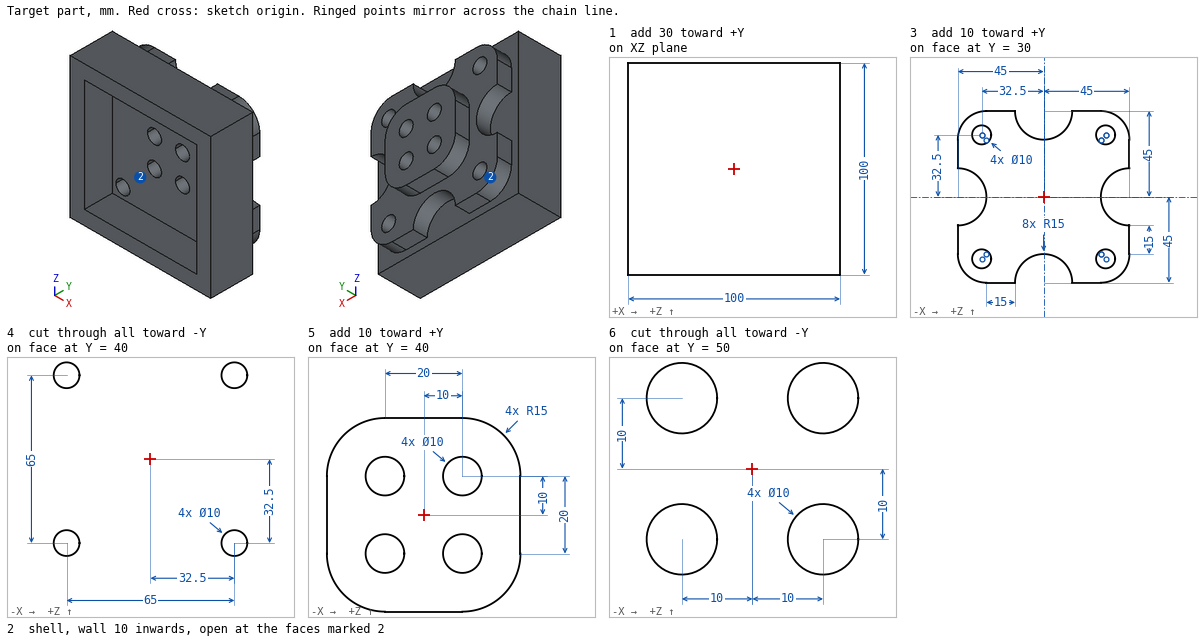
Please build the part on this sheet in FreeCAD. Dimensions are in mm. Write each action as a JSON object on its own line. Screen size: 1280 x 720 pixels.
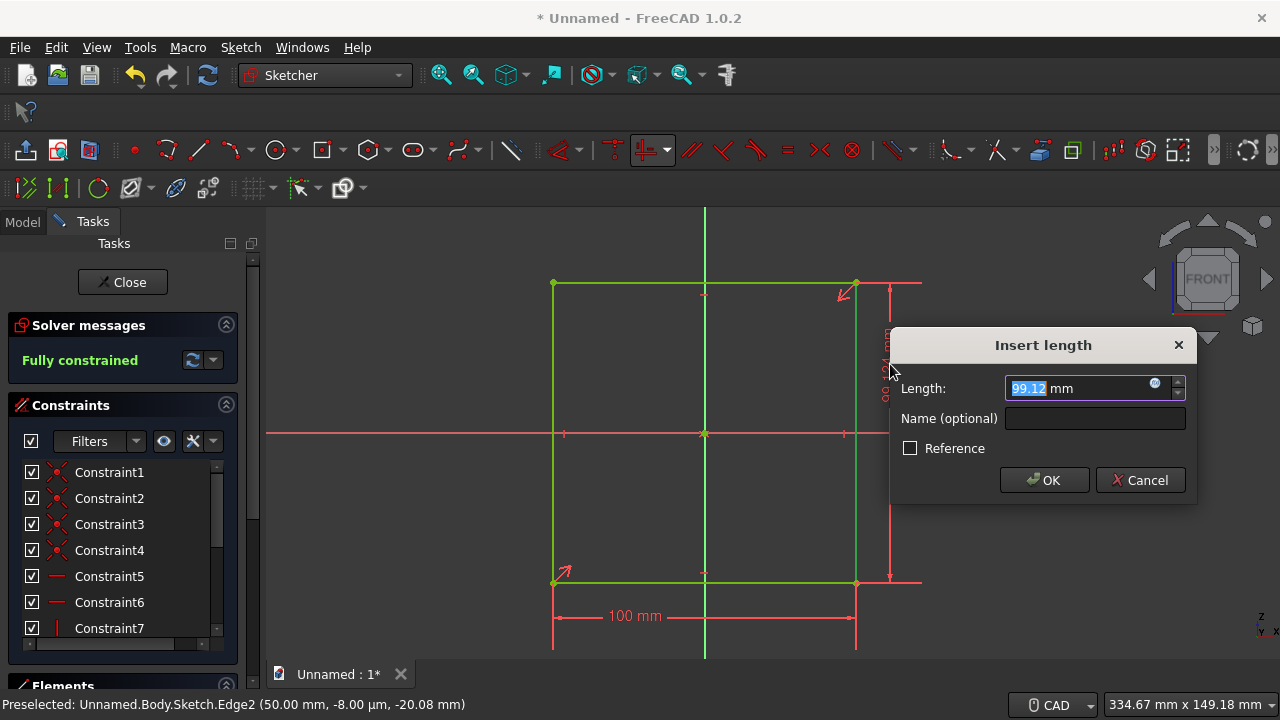
{"action": "type", "text": "100"}
{"action": "key", "text": "Return"}
{"action": "key", "text": "Escape"}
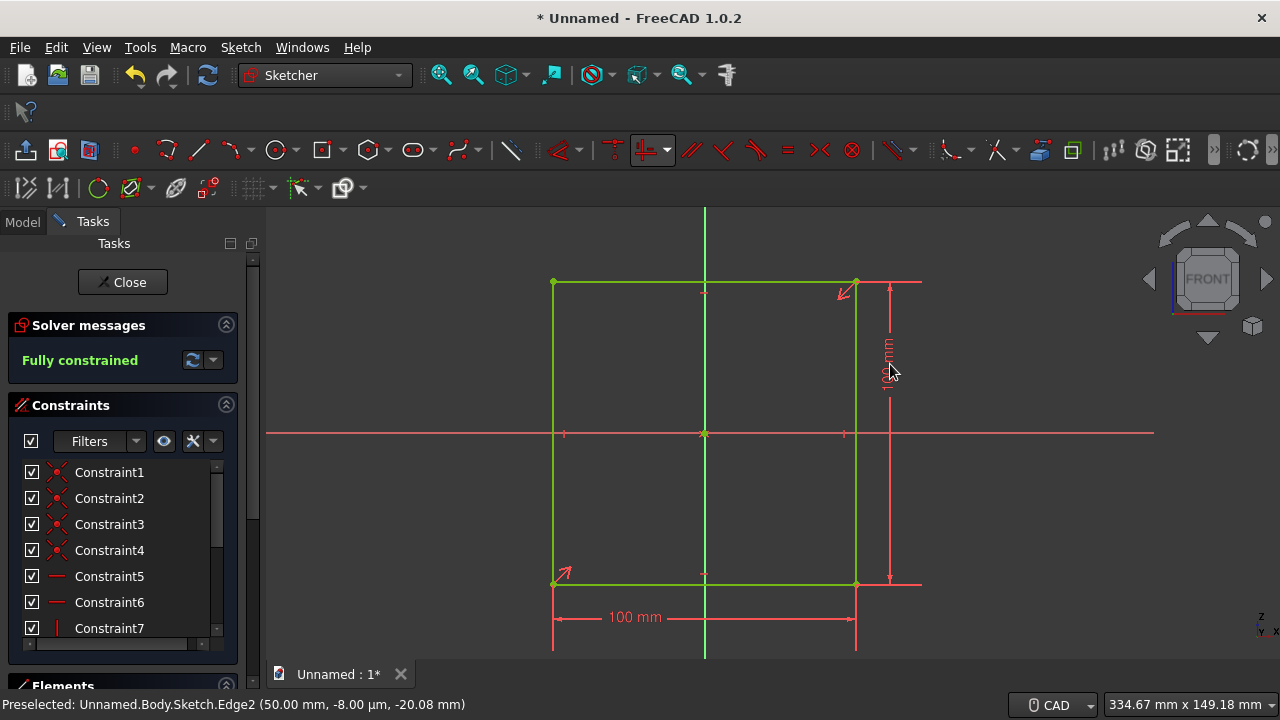
{"action": "left_click", "coordinate": [123, 282]}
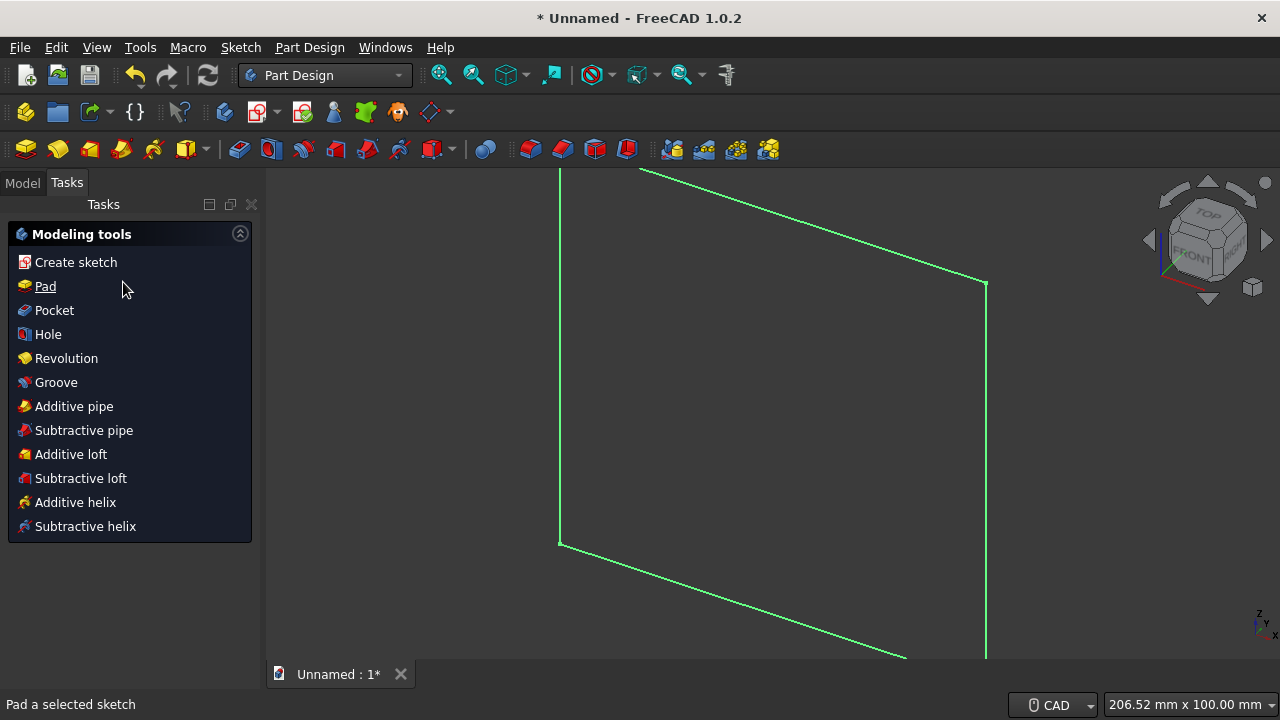
{"action": "left_click", "coordinate": [26, 150]}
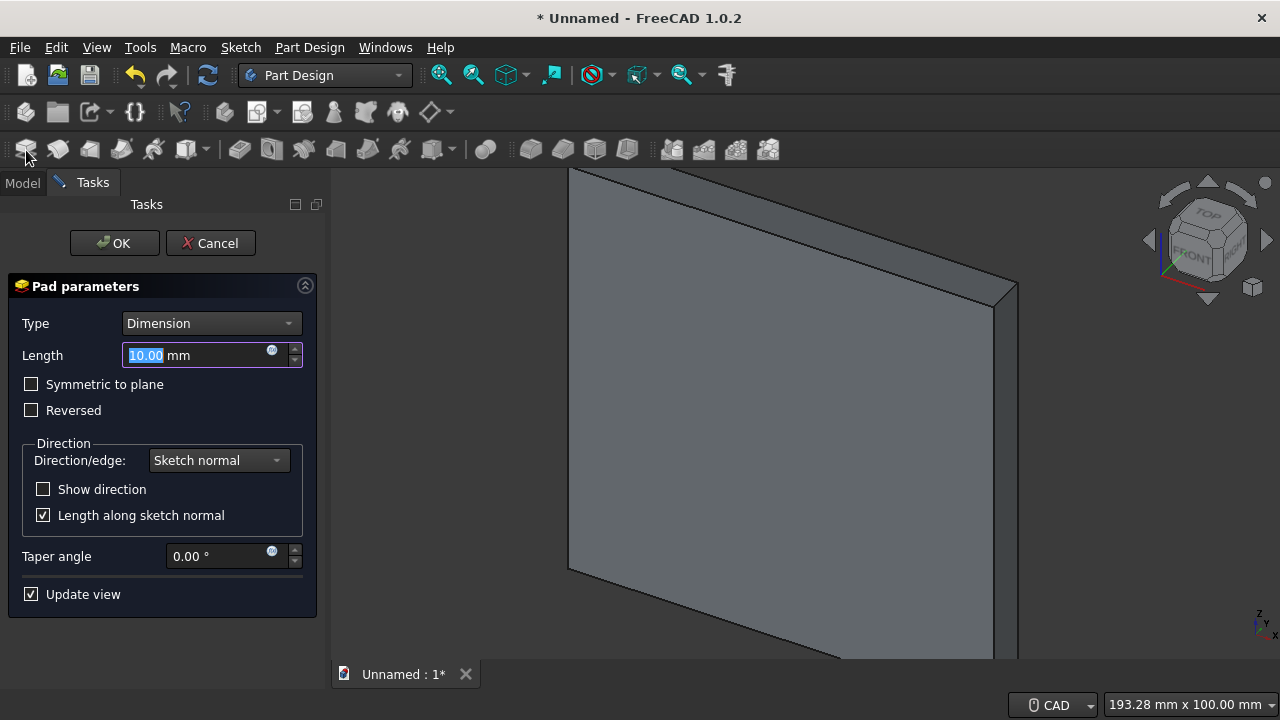
{"action": "type", "text": "30"}
{"action": "key", "text": "Tab"}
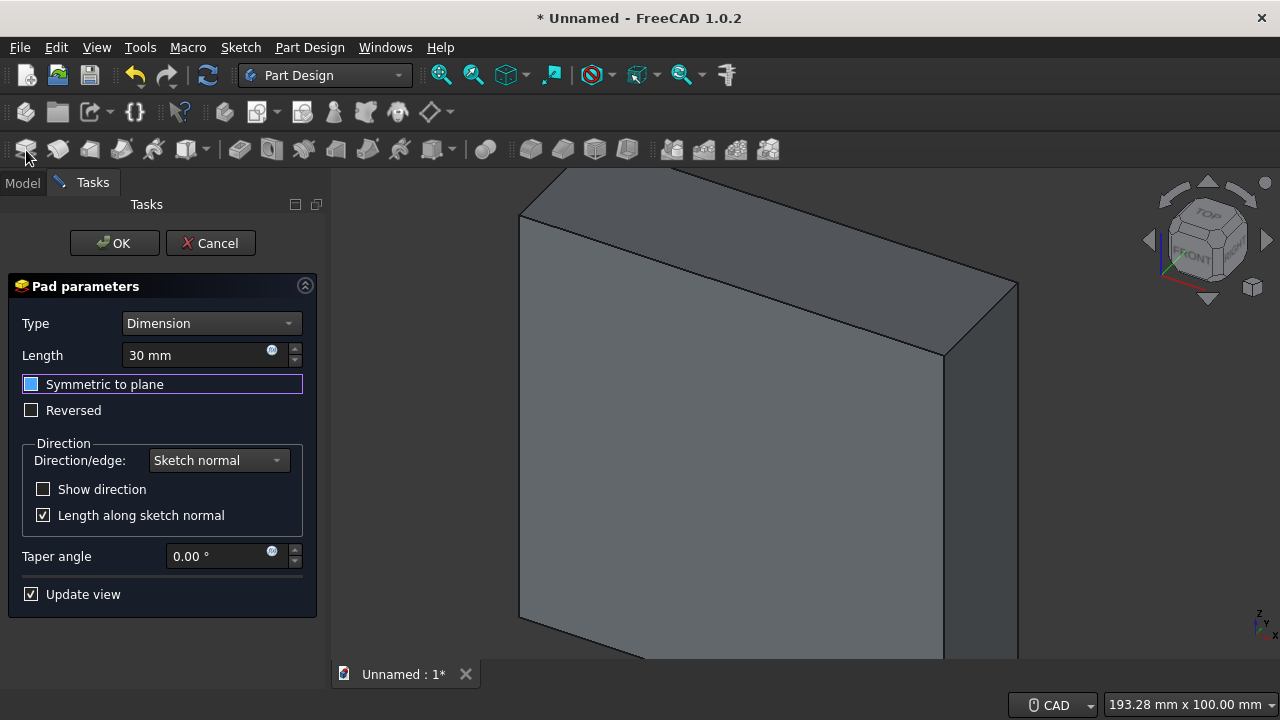
{"action": "left_click", "coordinate": [30, 410]}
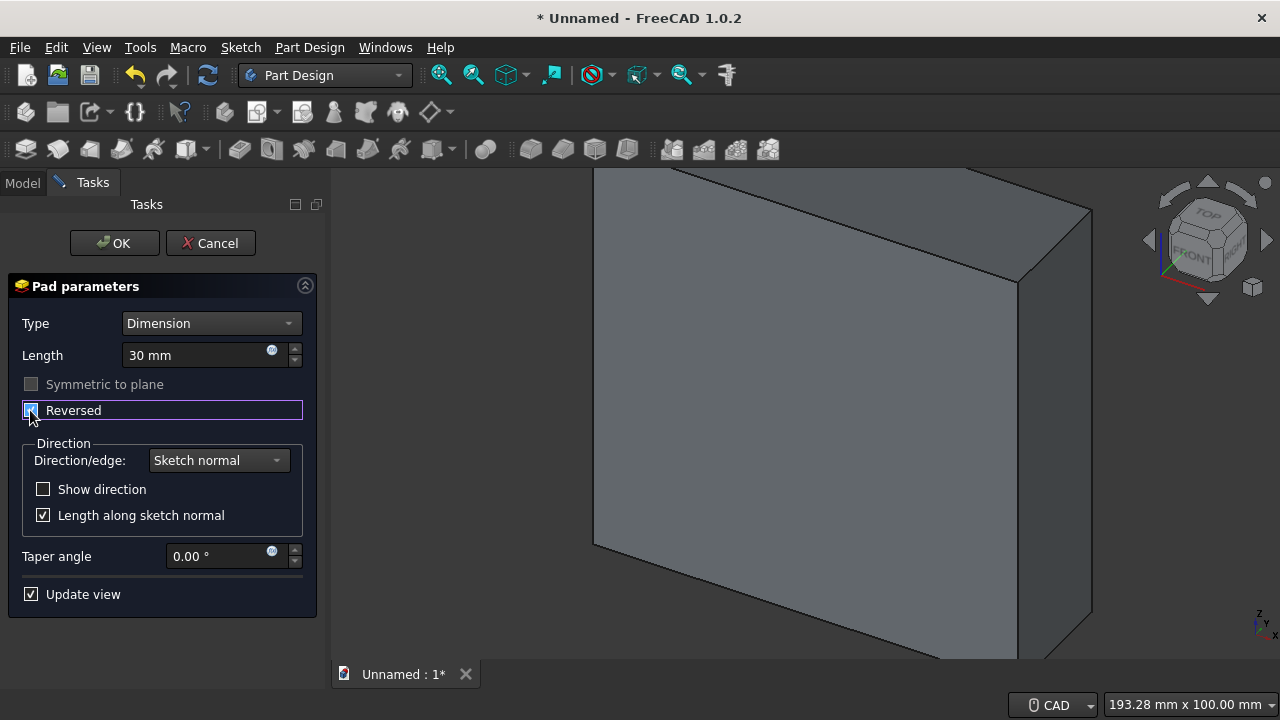
{"action": "left_click", "coordinate": [115, 243]}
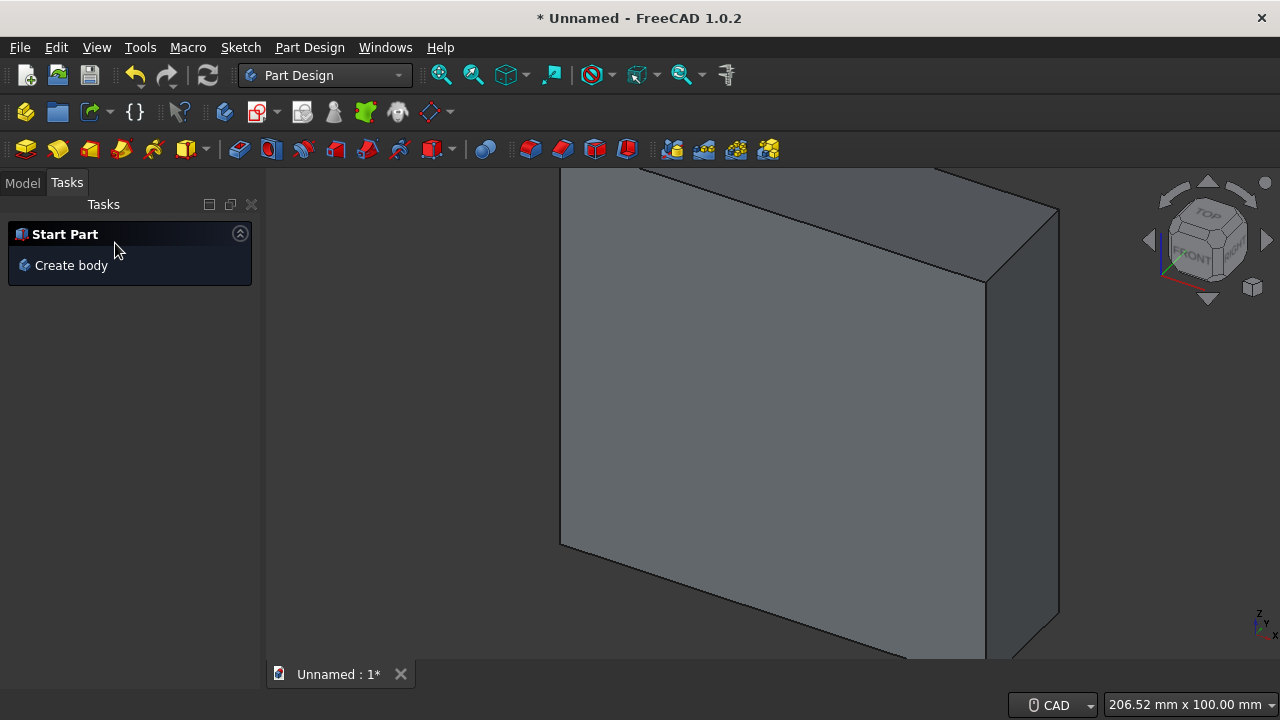
{"action": "left_click", "coordinate": [442, 76]}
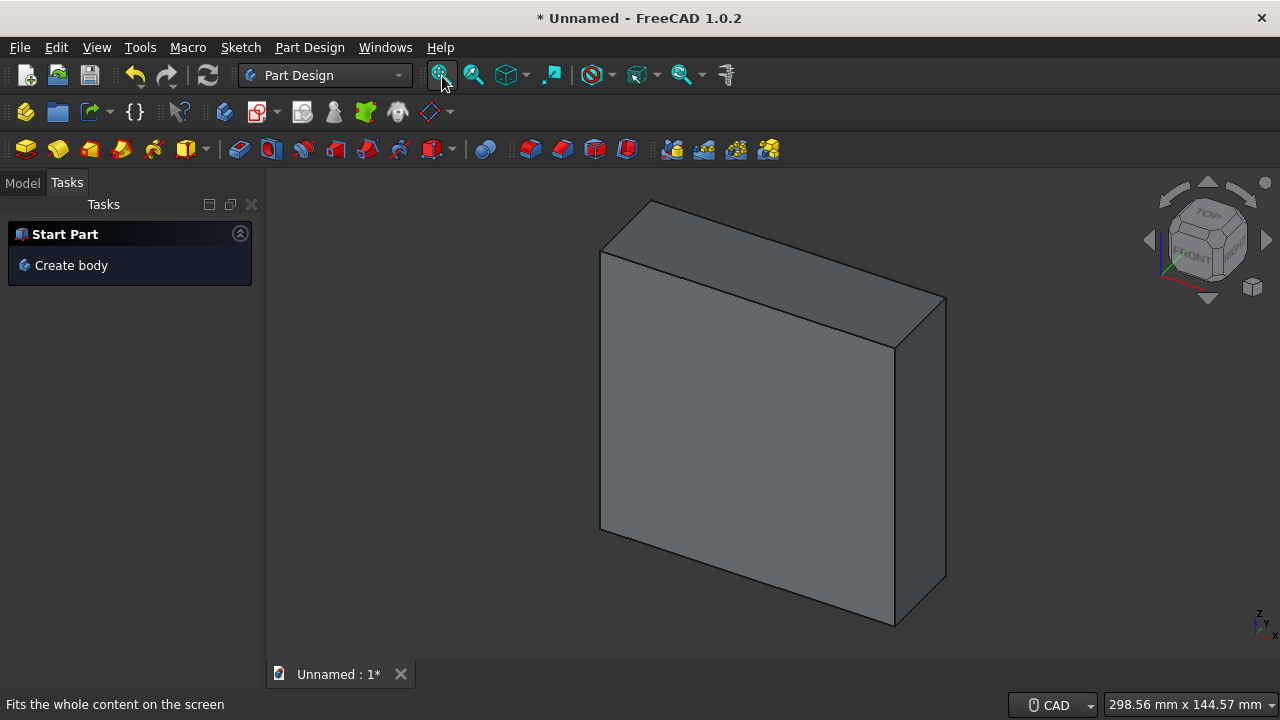
{"action": "left_click", "coordinate": [748, 438]}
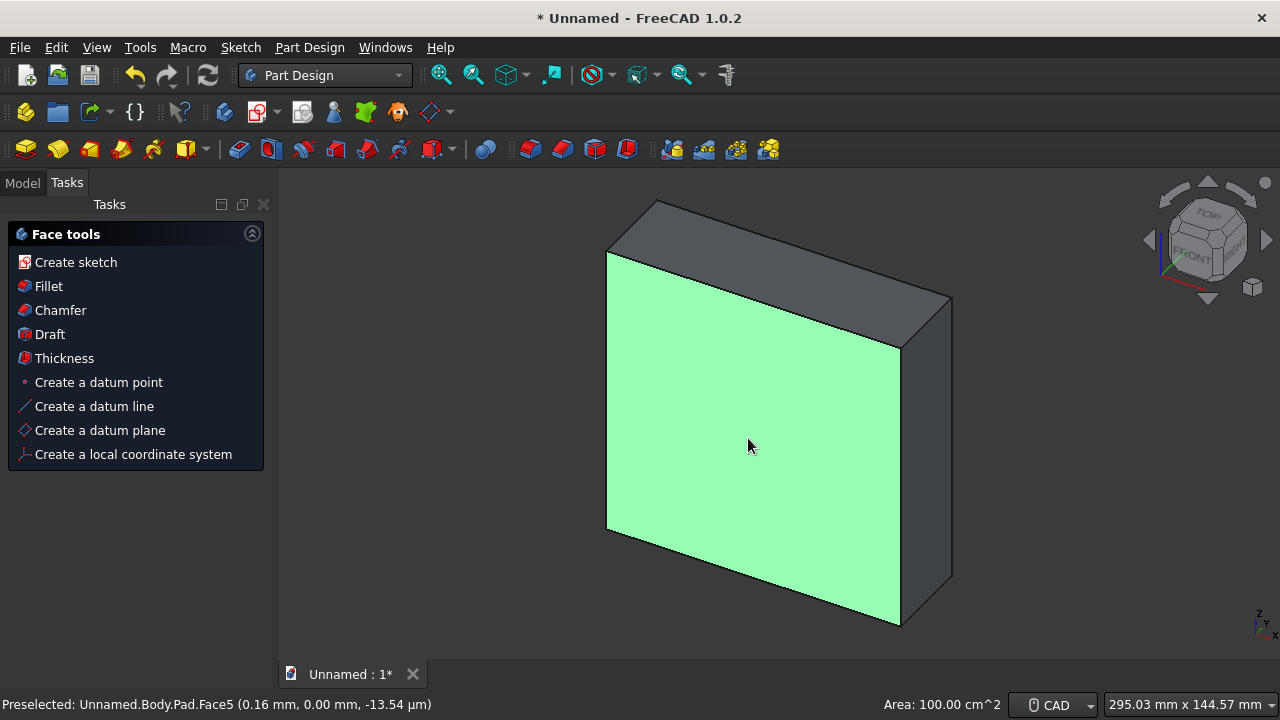
{"action": "left_click", "coordinate": [628, 150]}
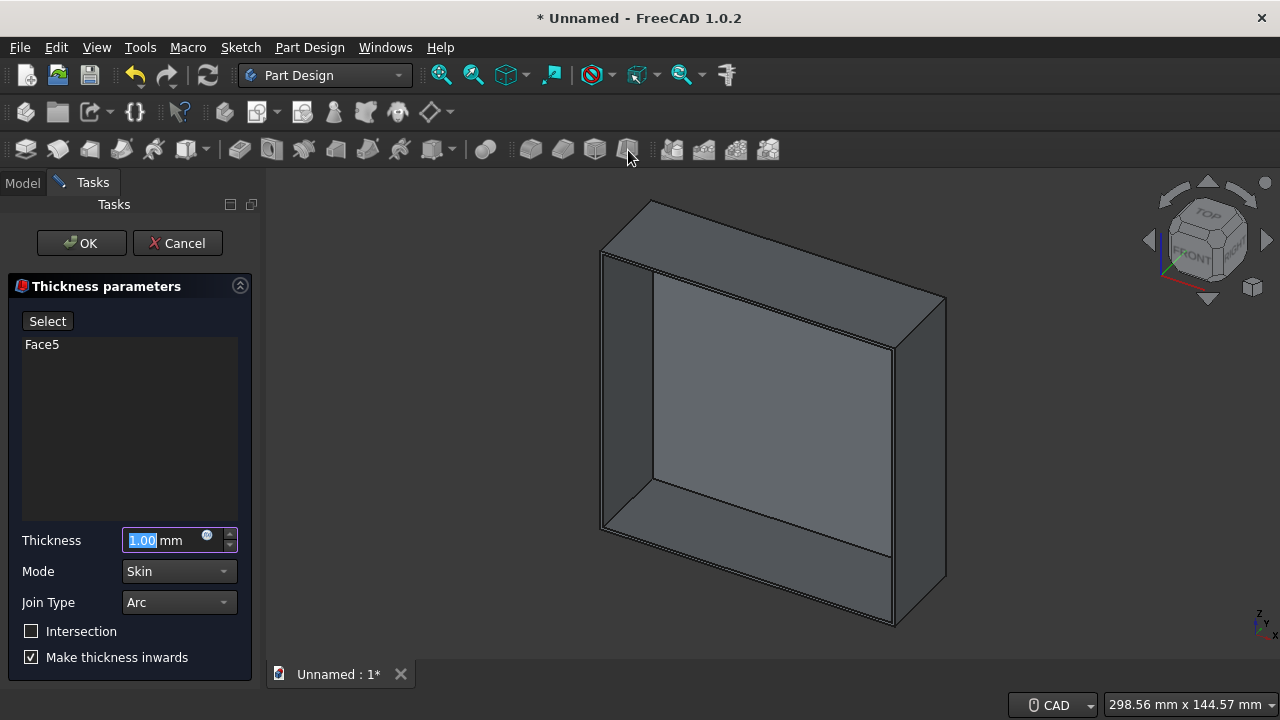
{"action": "type", "text": "10"}
{"action": "key", "text": "Tab"}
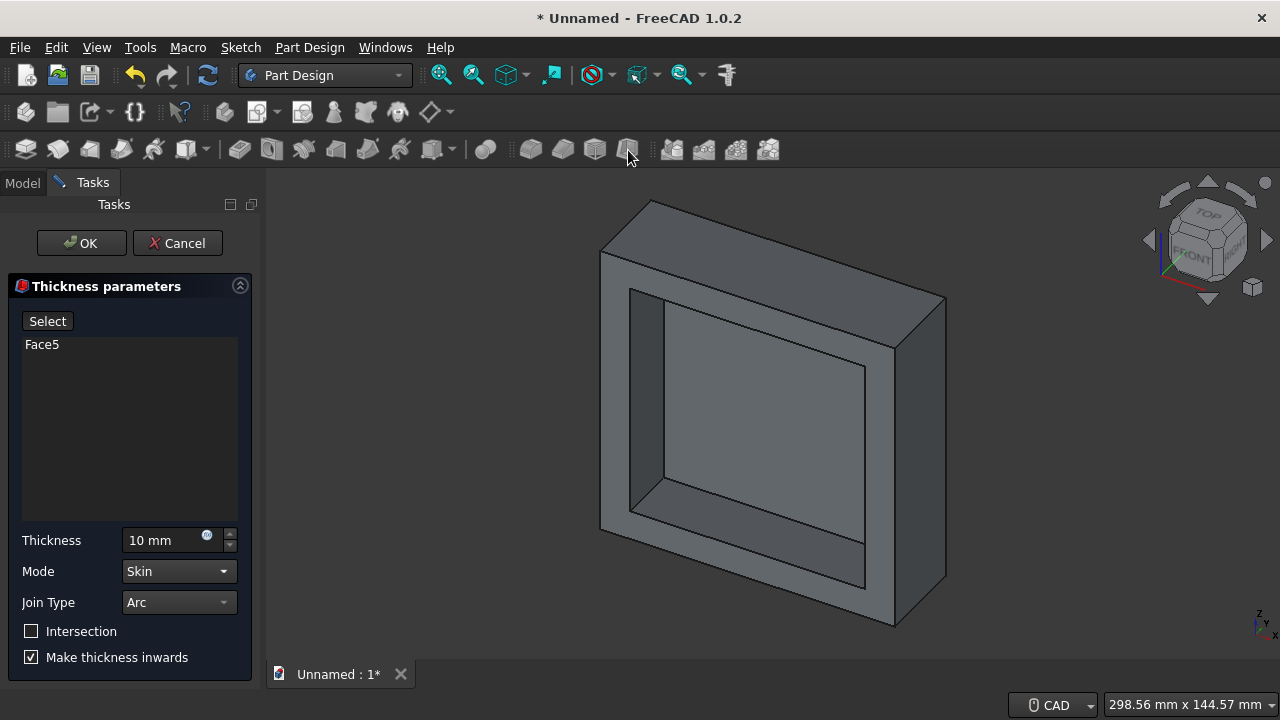
{"action": "left_click", "coordinate": [180, 602]}